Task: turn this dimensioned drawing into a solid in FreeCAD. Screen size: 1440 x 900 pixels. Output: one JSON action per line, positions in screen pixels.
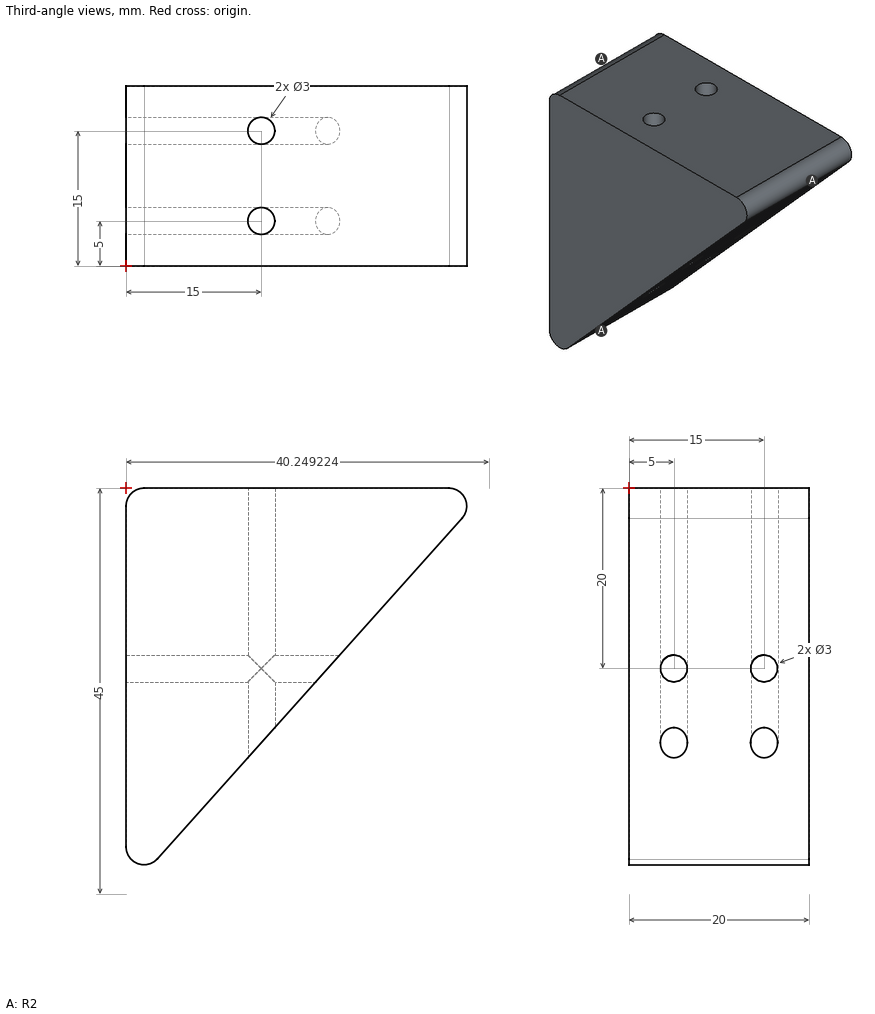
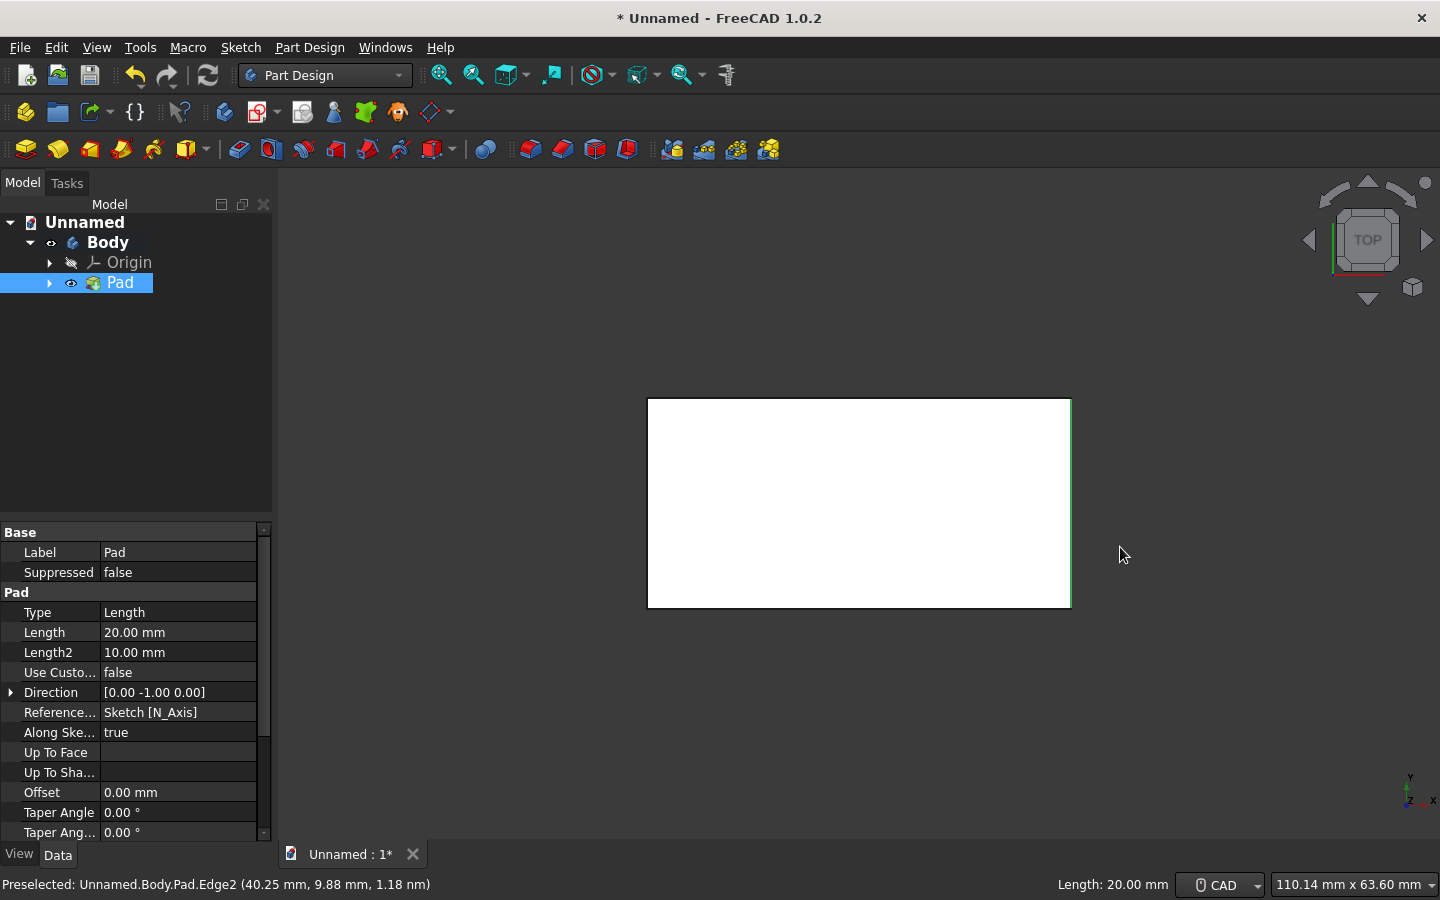
{"action": "key", "text": "v f"}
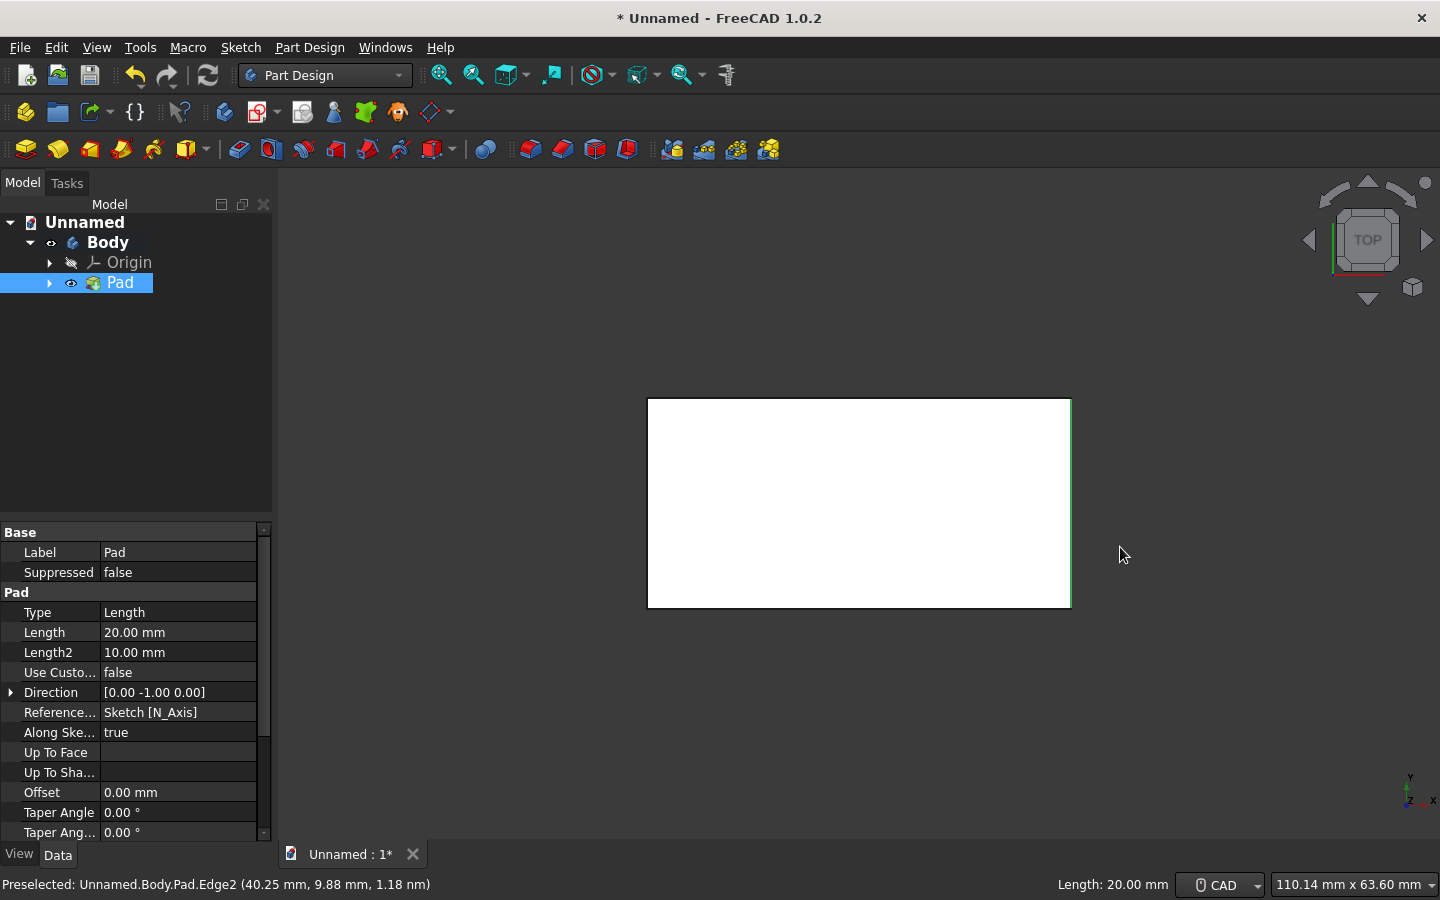
{"action": "left_click", "coordinate": [647, 503], "text": "ctrl"}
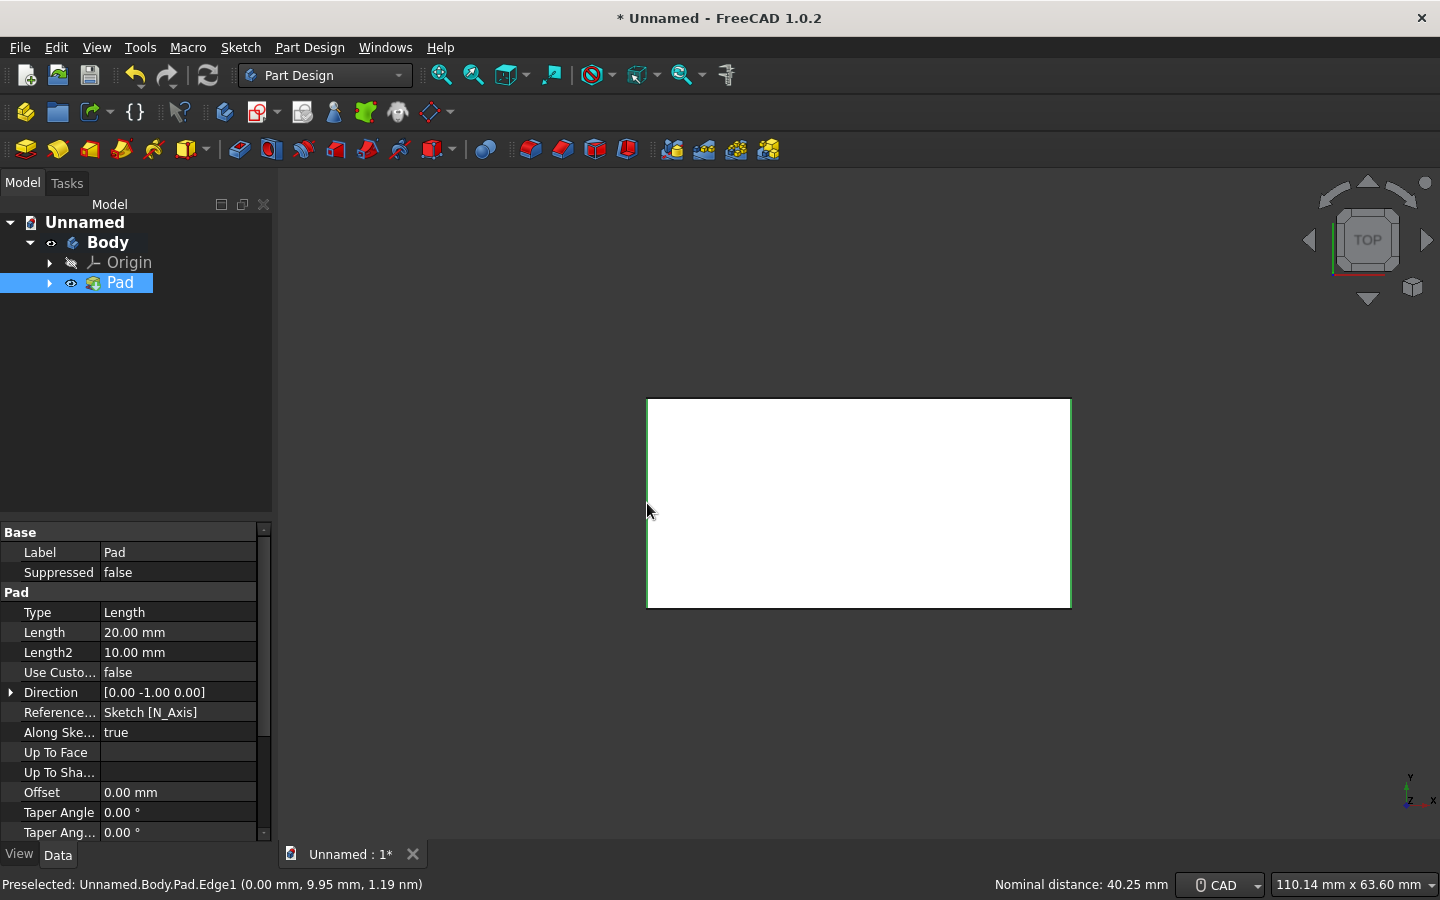
{"action": "key", "text": "1"}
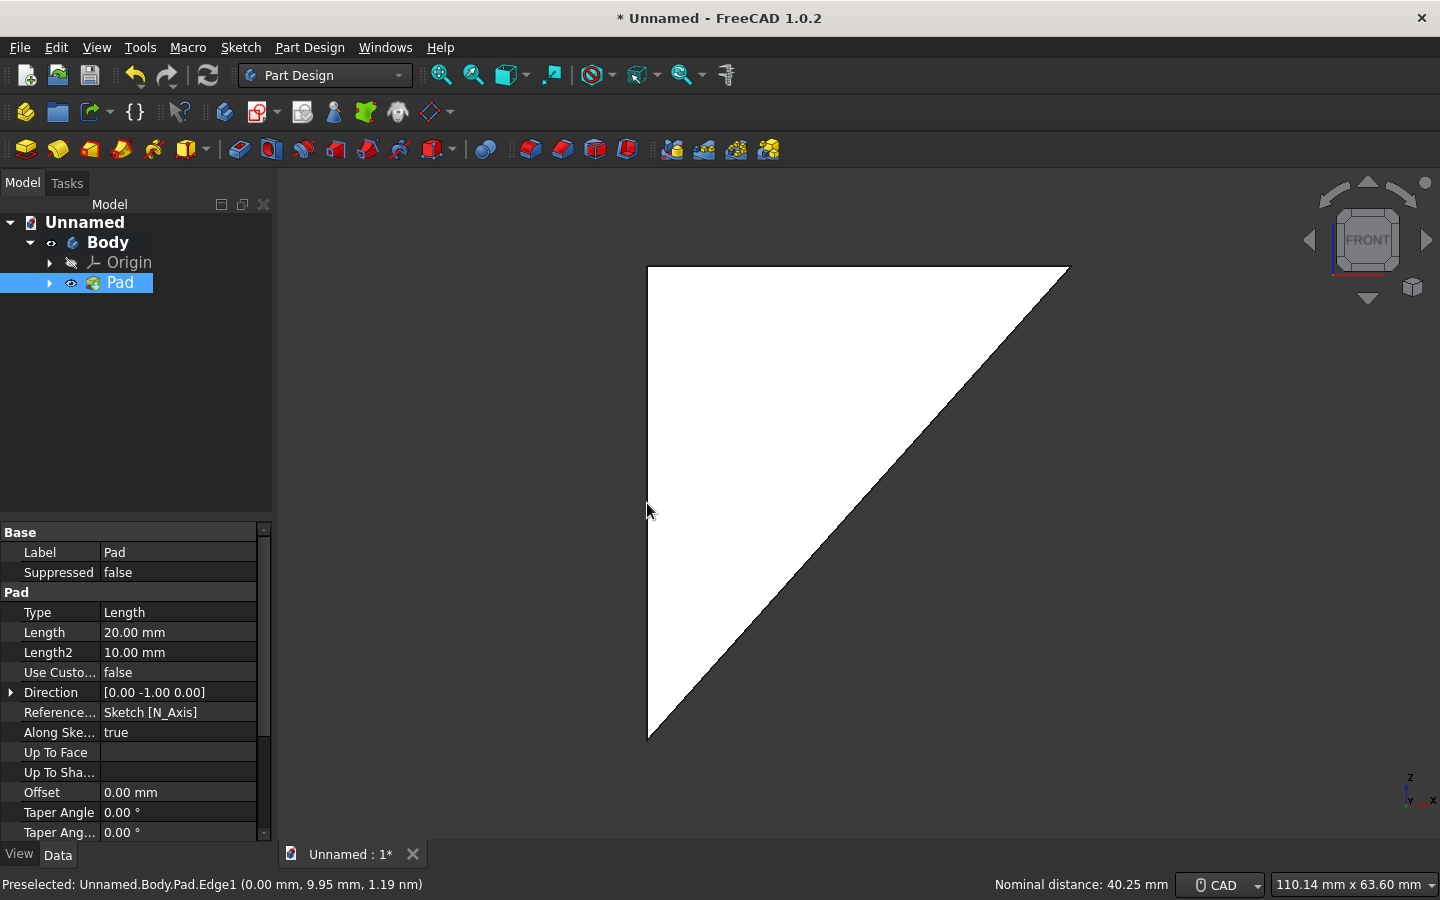
{"action": "key", "text": "3"}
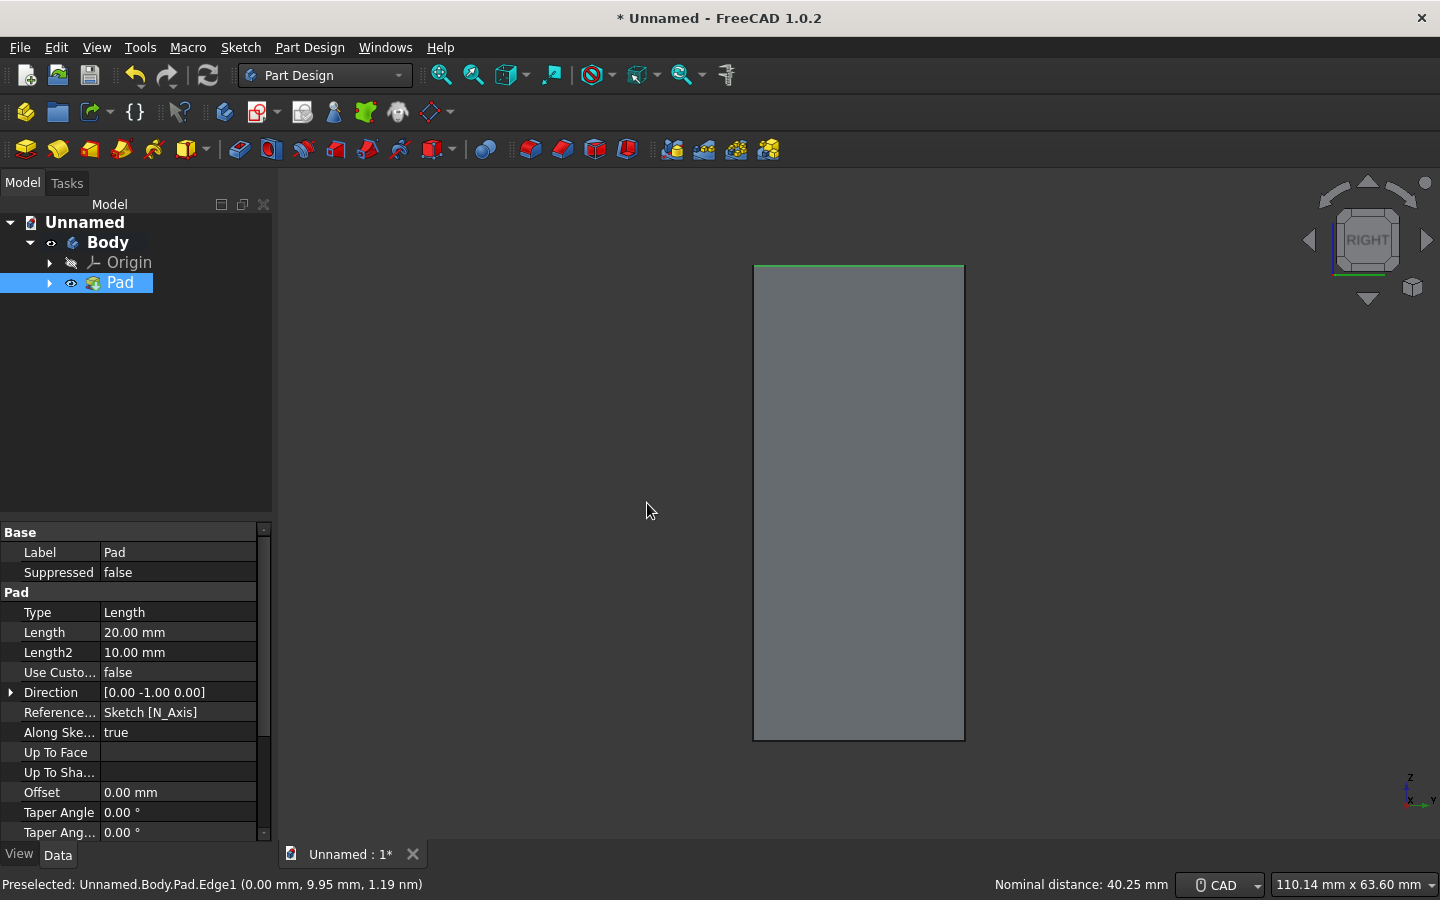
{"action": "key", "text": "5"}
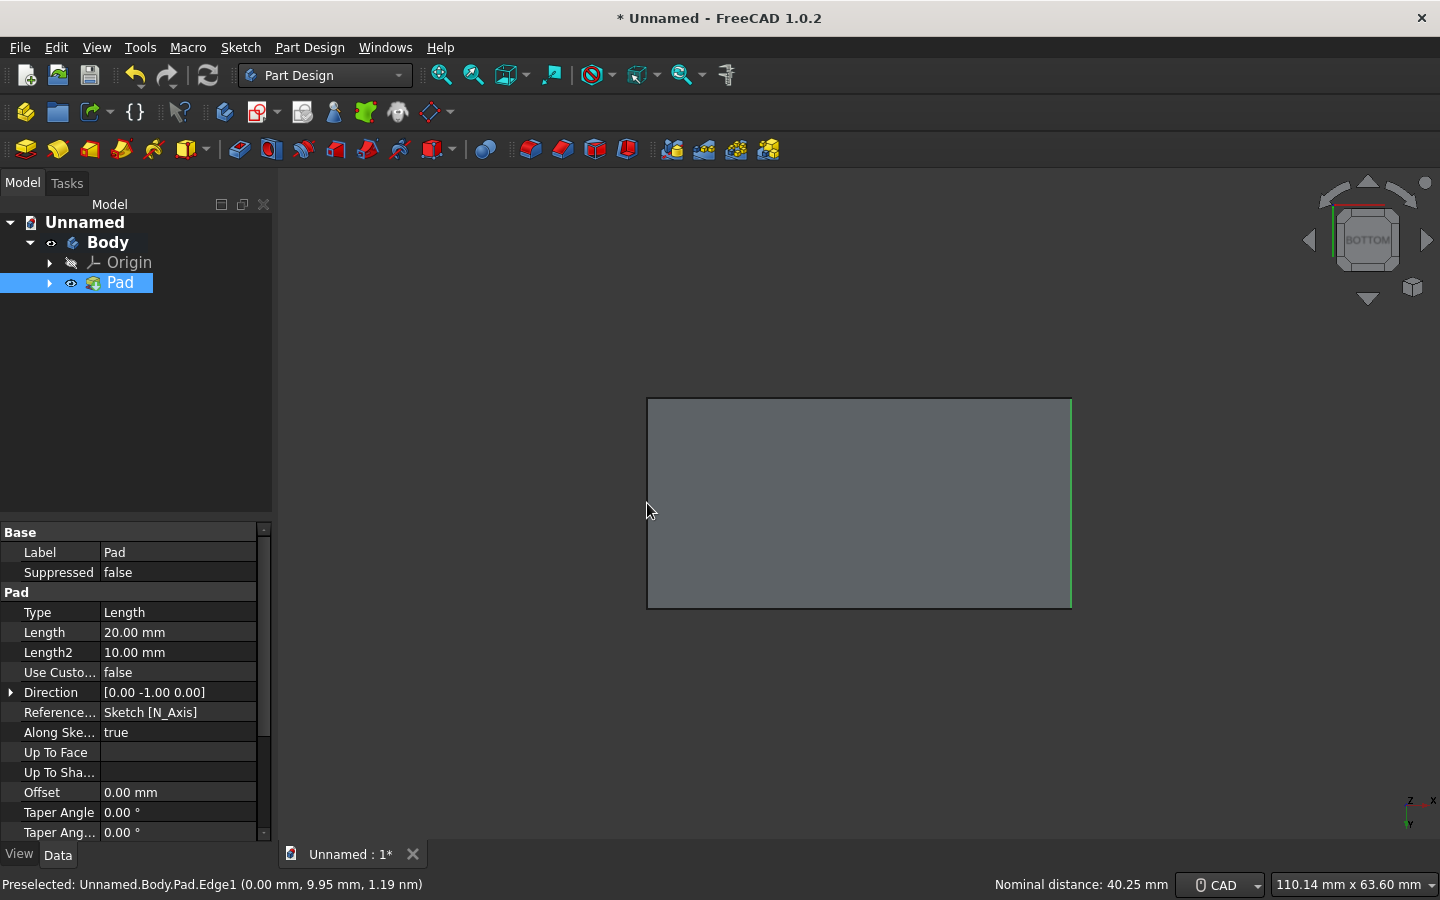
{"action": "left_click", "coordinate": [442, 76]}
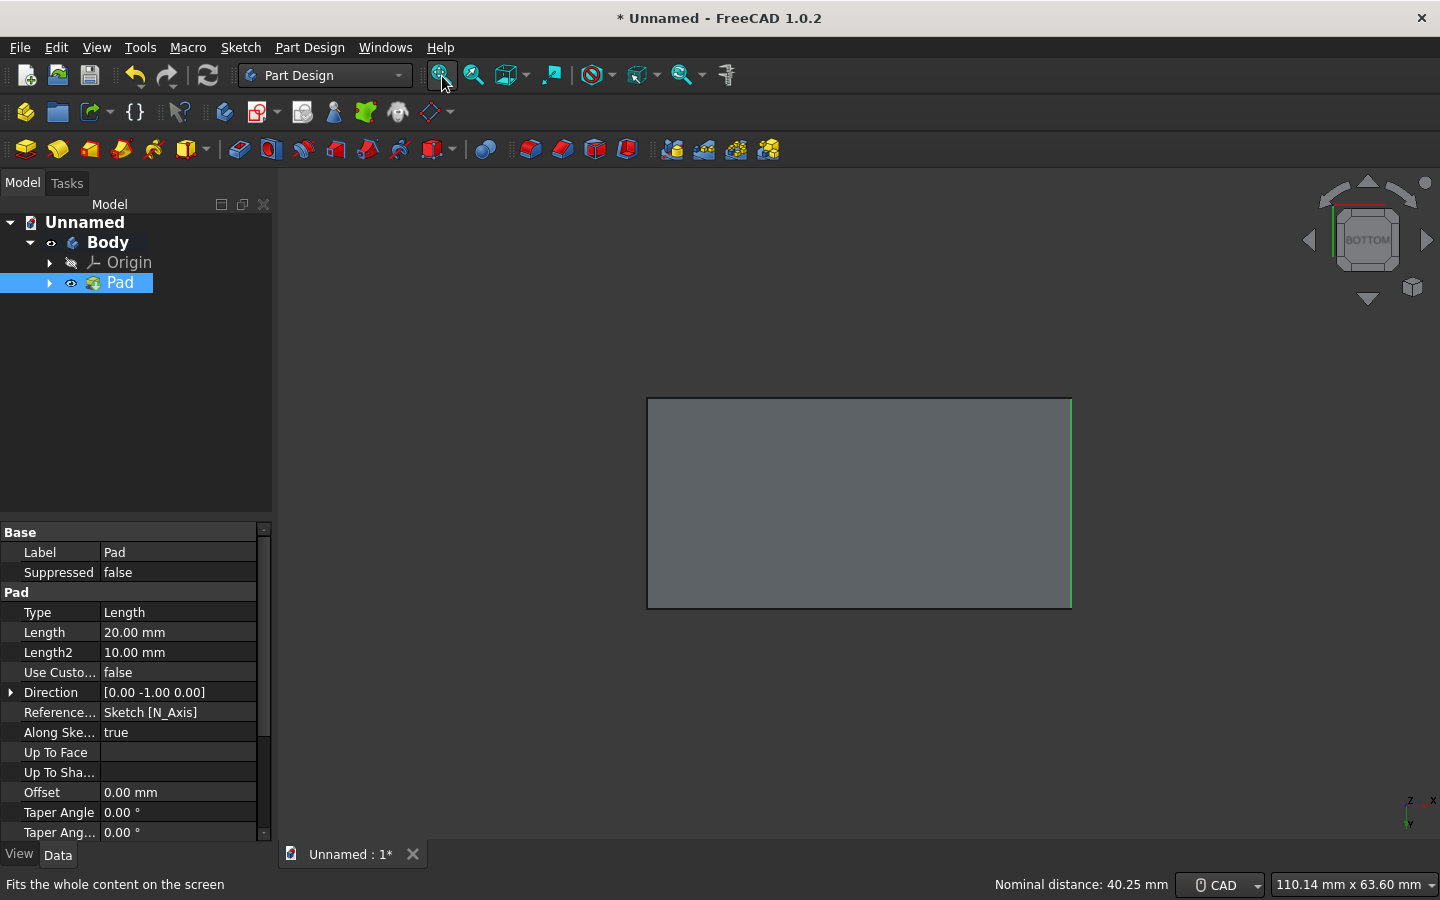
{"action": "left_click", "coordinate": [647, 502], "text": "ctrl"}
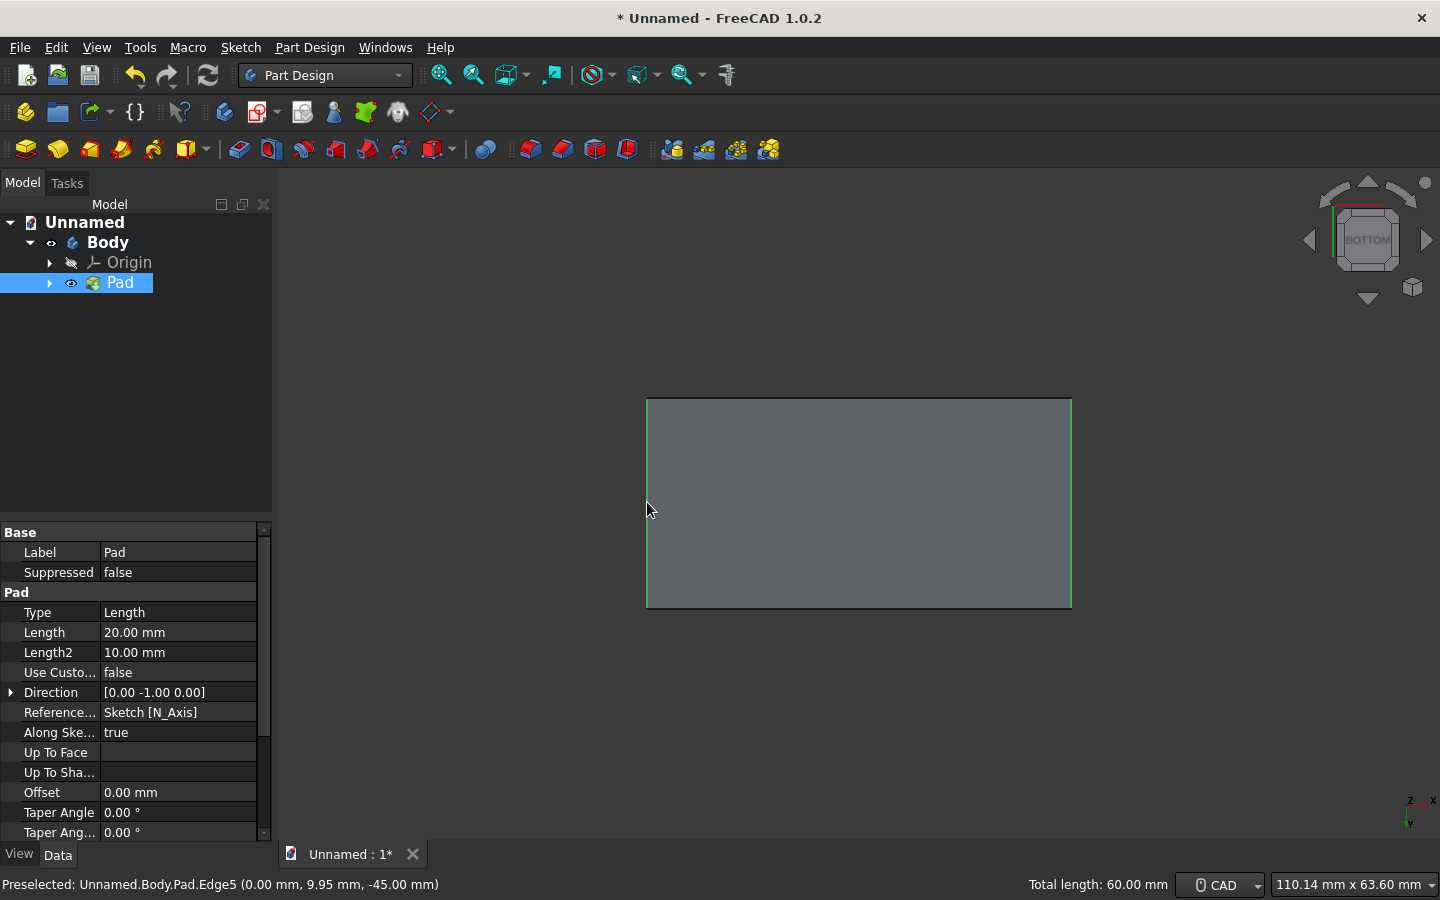
{"action": "left_click", "coordinate": [532, 150]}